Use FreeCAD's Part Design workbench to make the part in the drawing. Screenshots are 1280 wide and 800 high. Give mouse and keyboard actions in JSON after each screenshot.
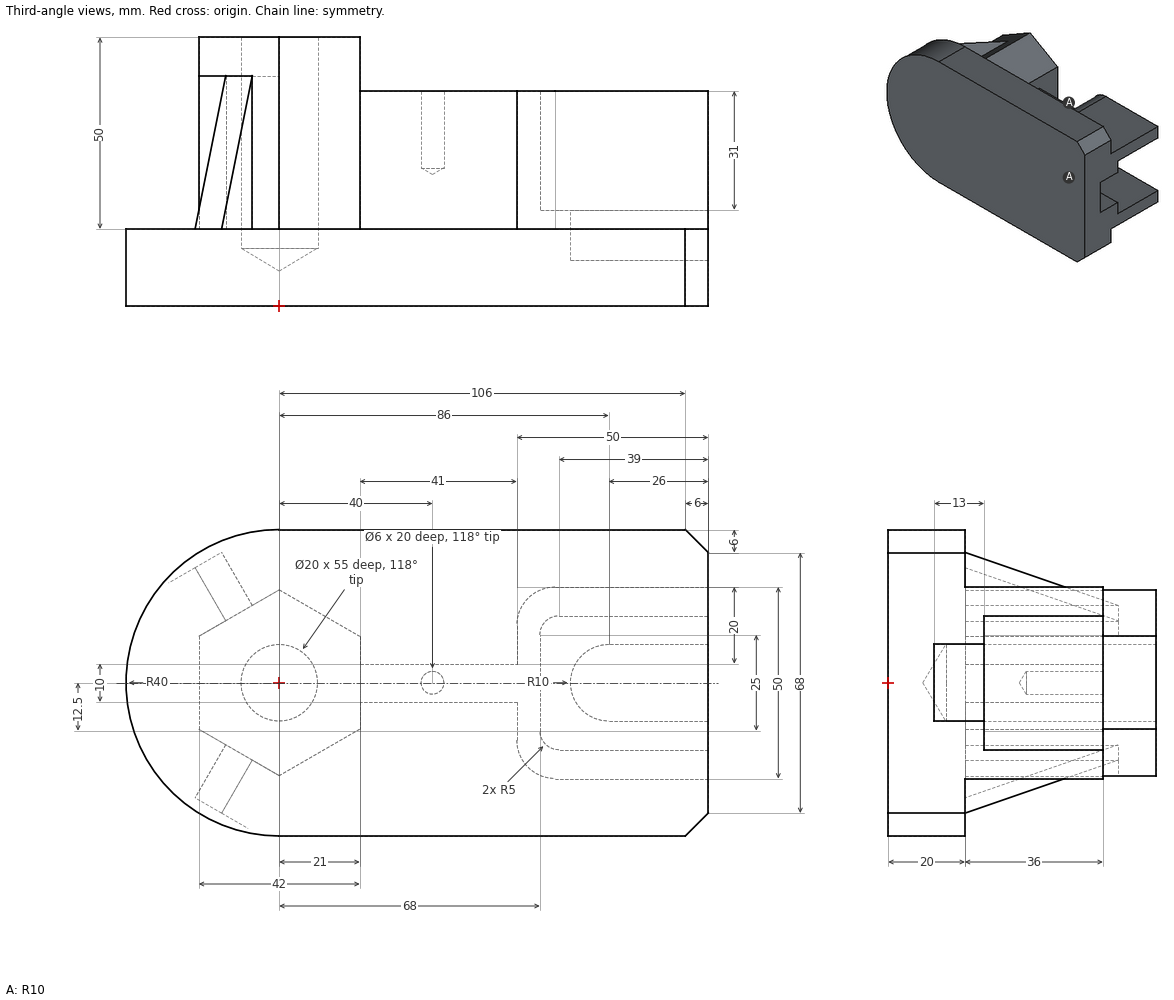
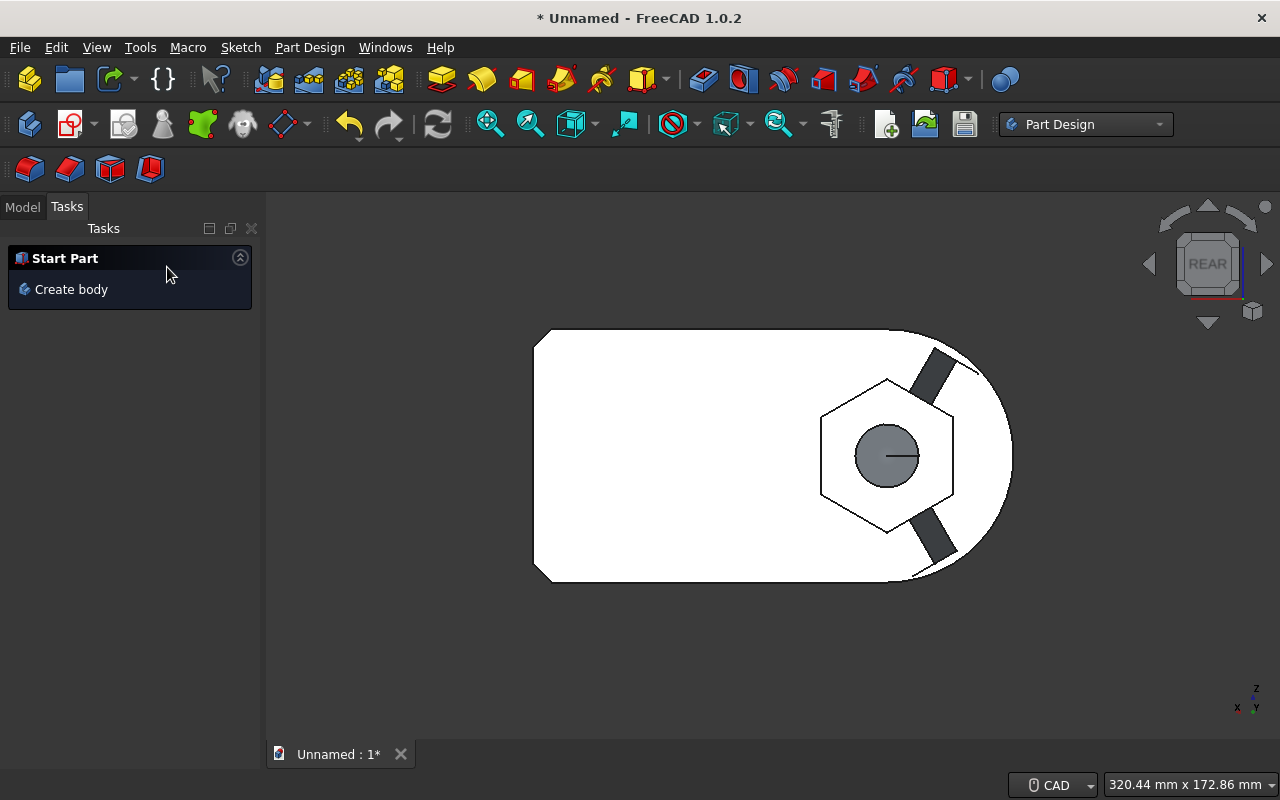
{"action": "left_click", "coordinate": [704, 455]}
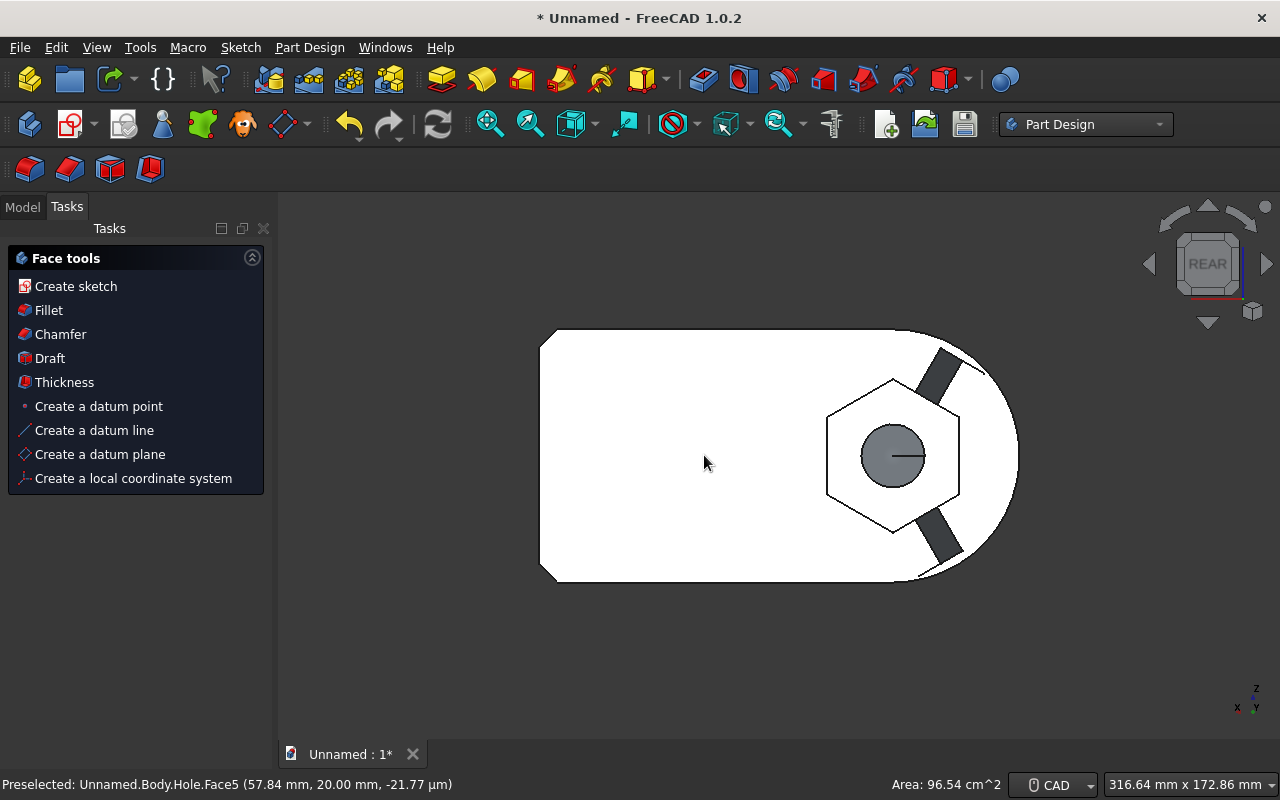
{"action": "left_click", "coordinate": [70, 124]}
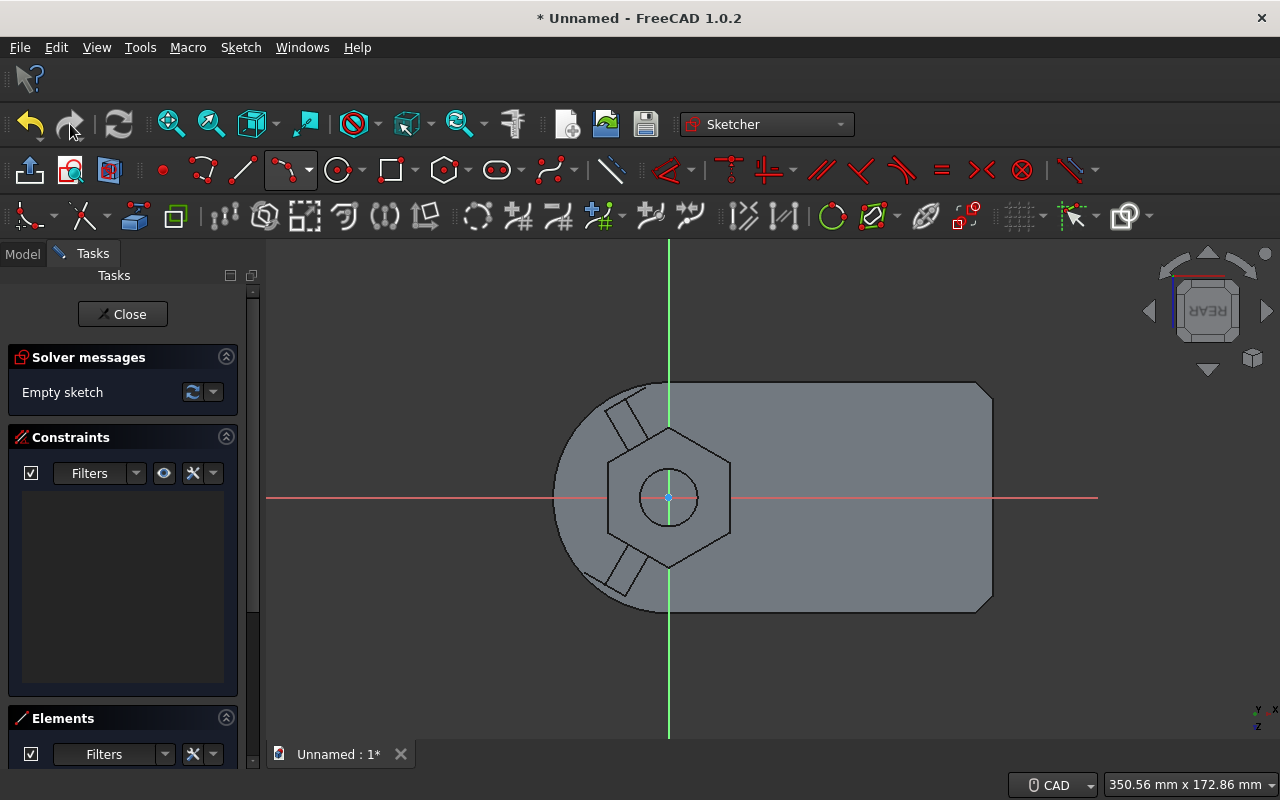
{"action": "scroll", "coordinate": [984, 508], "scroll_direction": "up", "scroll_amount": 3}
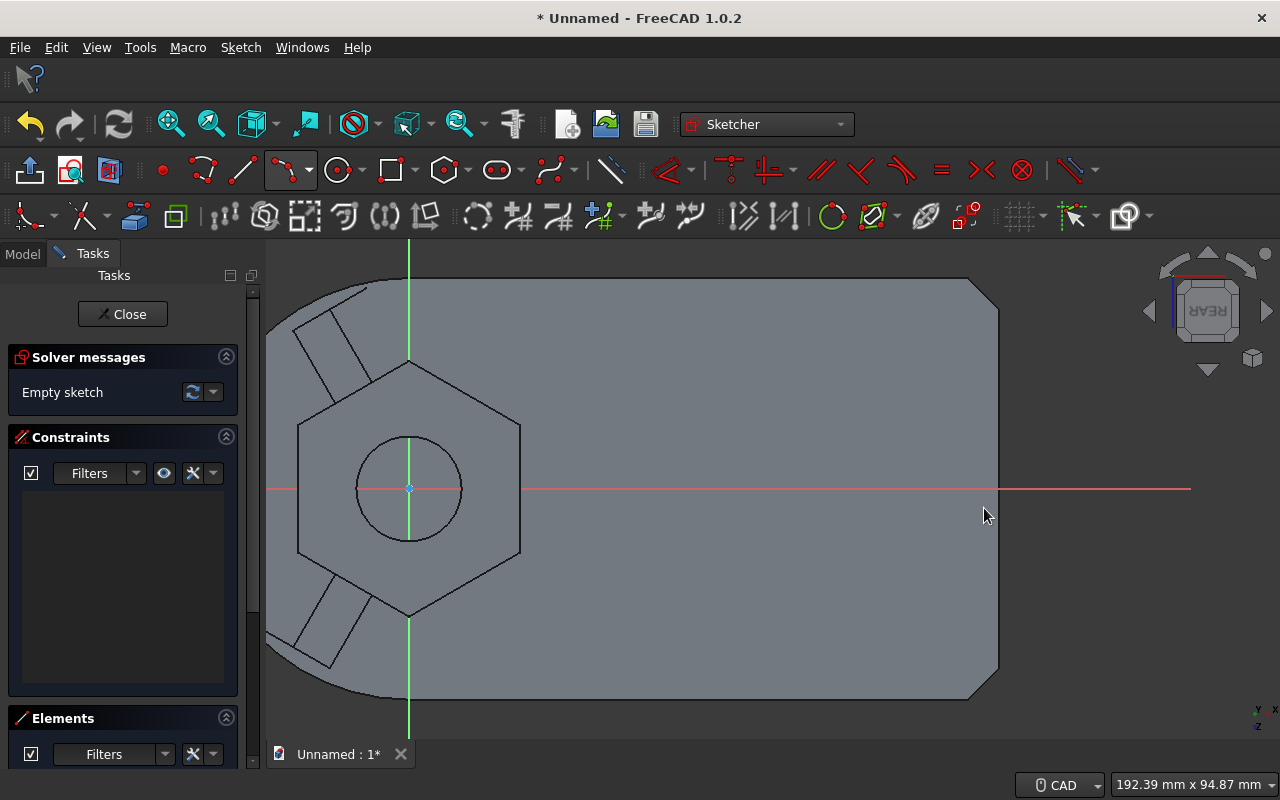
{"action": "left_click", "coordinate": [204, 170]}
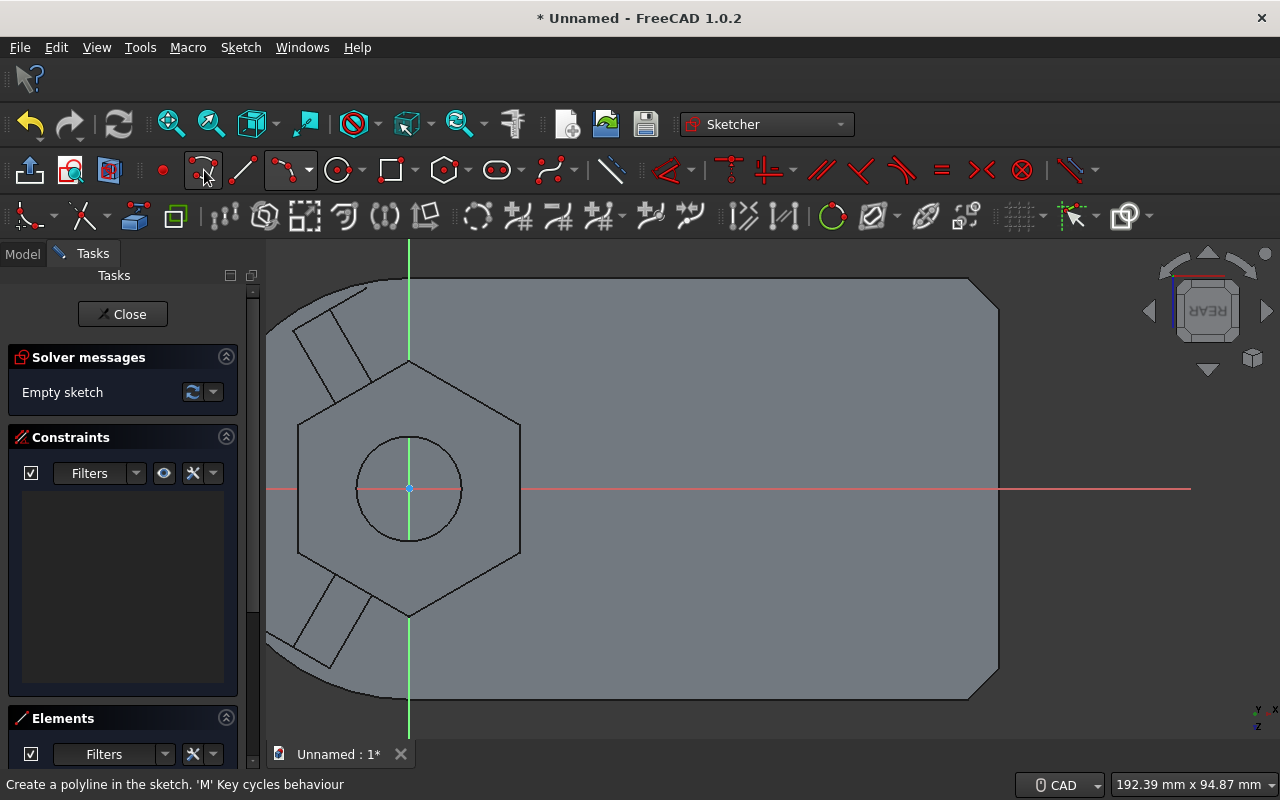
{"action": "left_click", "coordinate": [520, 463]}
{"action": "left_click", "coordinate": [520, 515]}
{"action": "left_click", "coordinate": [736, 515]}
{"action": "left_click", "coordinate": [736, 621]}
{"action": "left_click", "coordinate": [999, 621]}
{"action": "left_click", "coordinate": [999, 357]}
{"action": "left_click", "coordinate": [736, 357]}
{"action": "left_click", "coordinate": [736, 463]}
{"action": "left_click", "coordinate": [520, 464]}
{"action": "key", "text": "Escape"}
{"action": "key", "text": "Escape"}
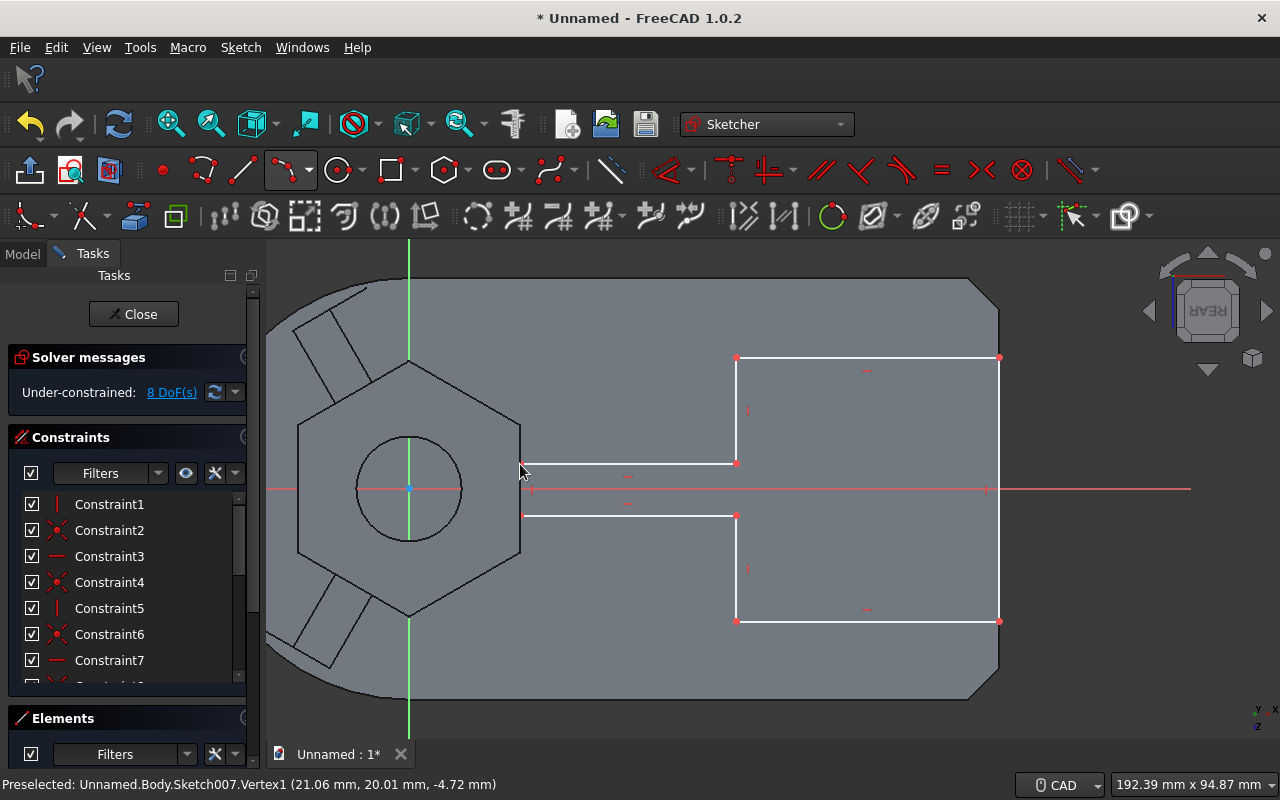
{"action": "left_click", "coordinate": [736, 622]}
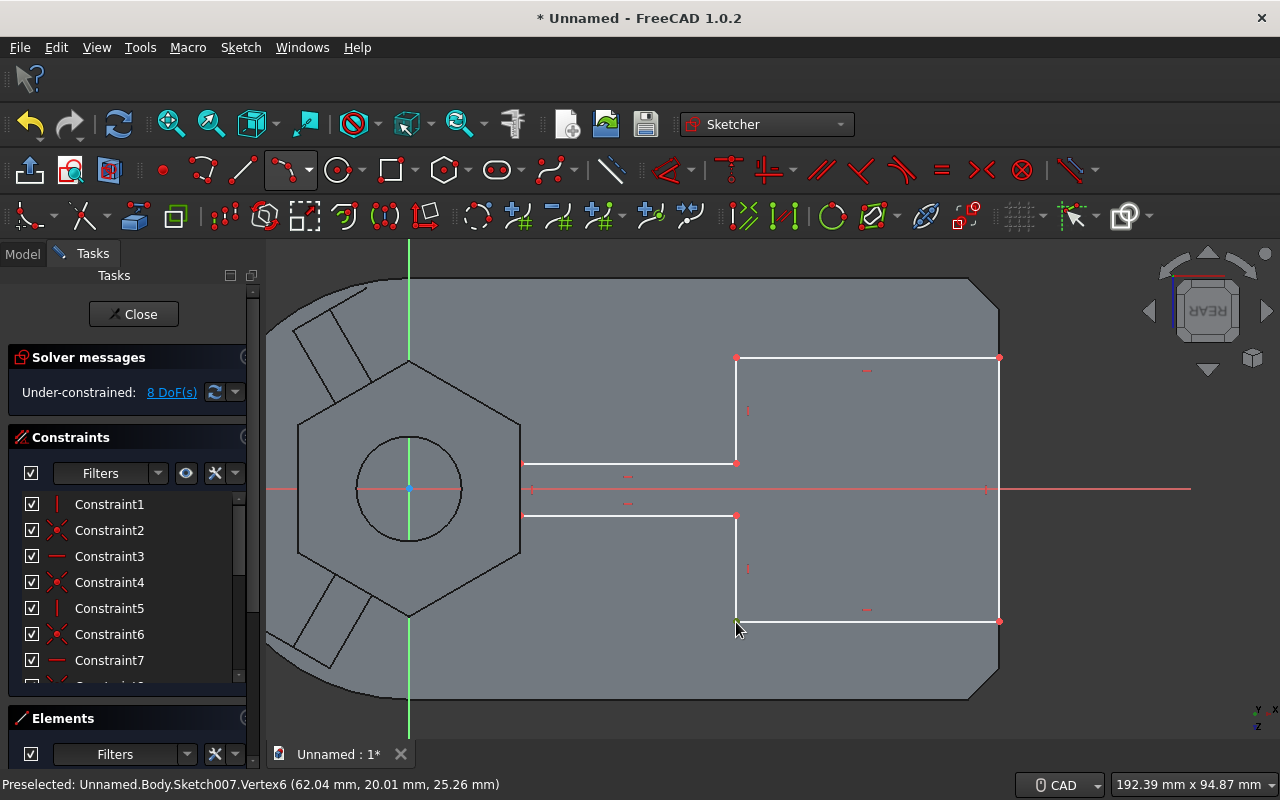
{"action": "left_click", "coordinate": [736, 358]}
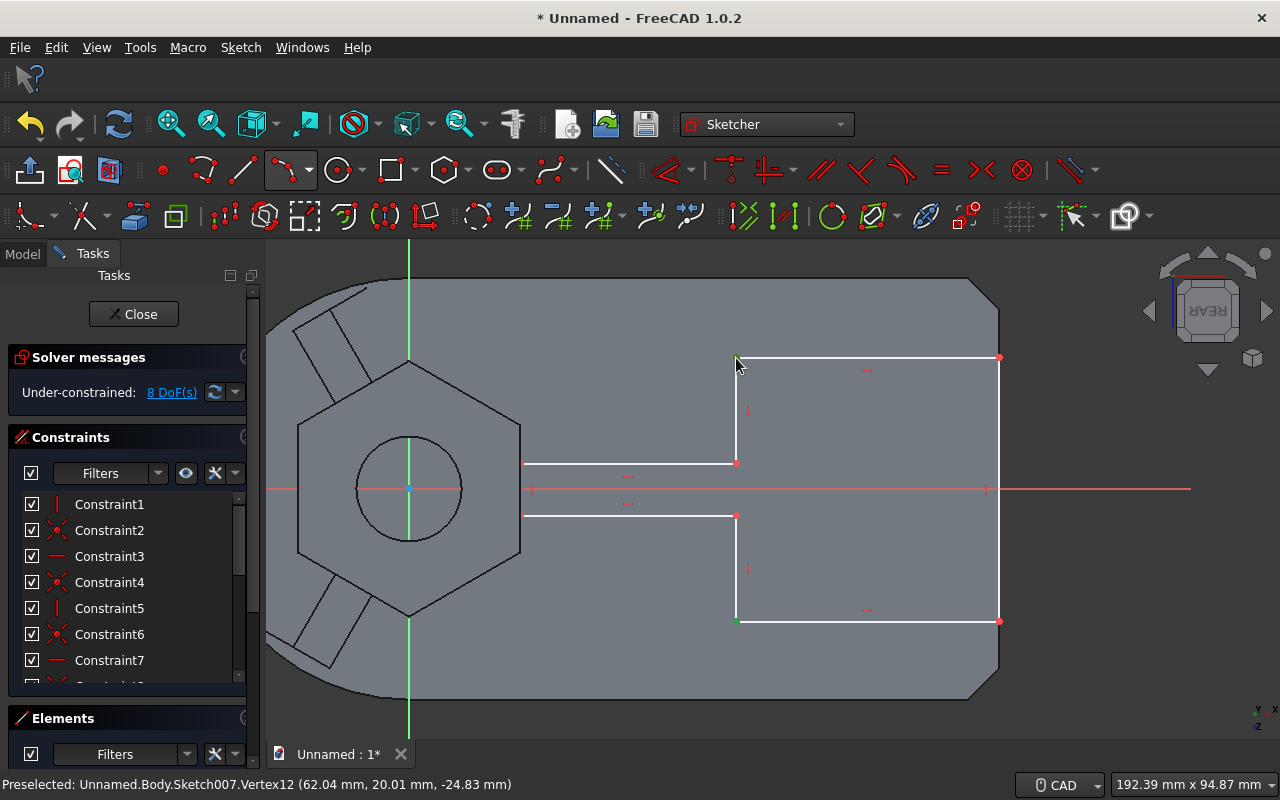
{"action": "left_click", "coordinate": [353, 489]}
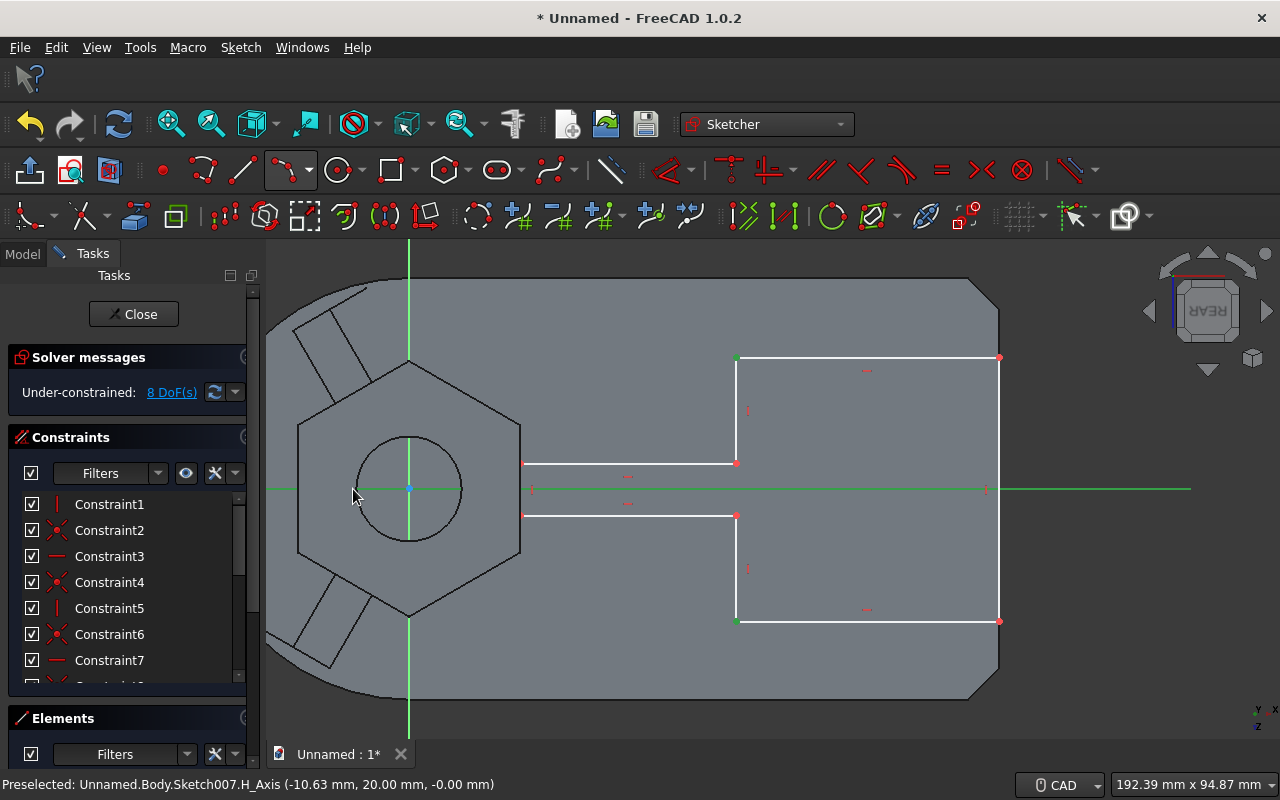
{"action": "left_click", "coordinate": [982, 170]}